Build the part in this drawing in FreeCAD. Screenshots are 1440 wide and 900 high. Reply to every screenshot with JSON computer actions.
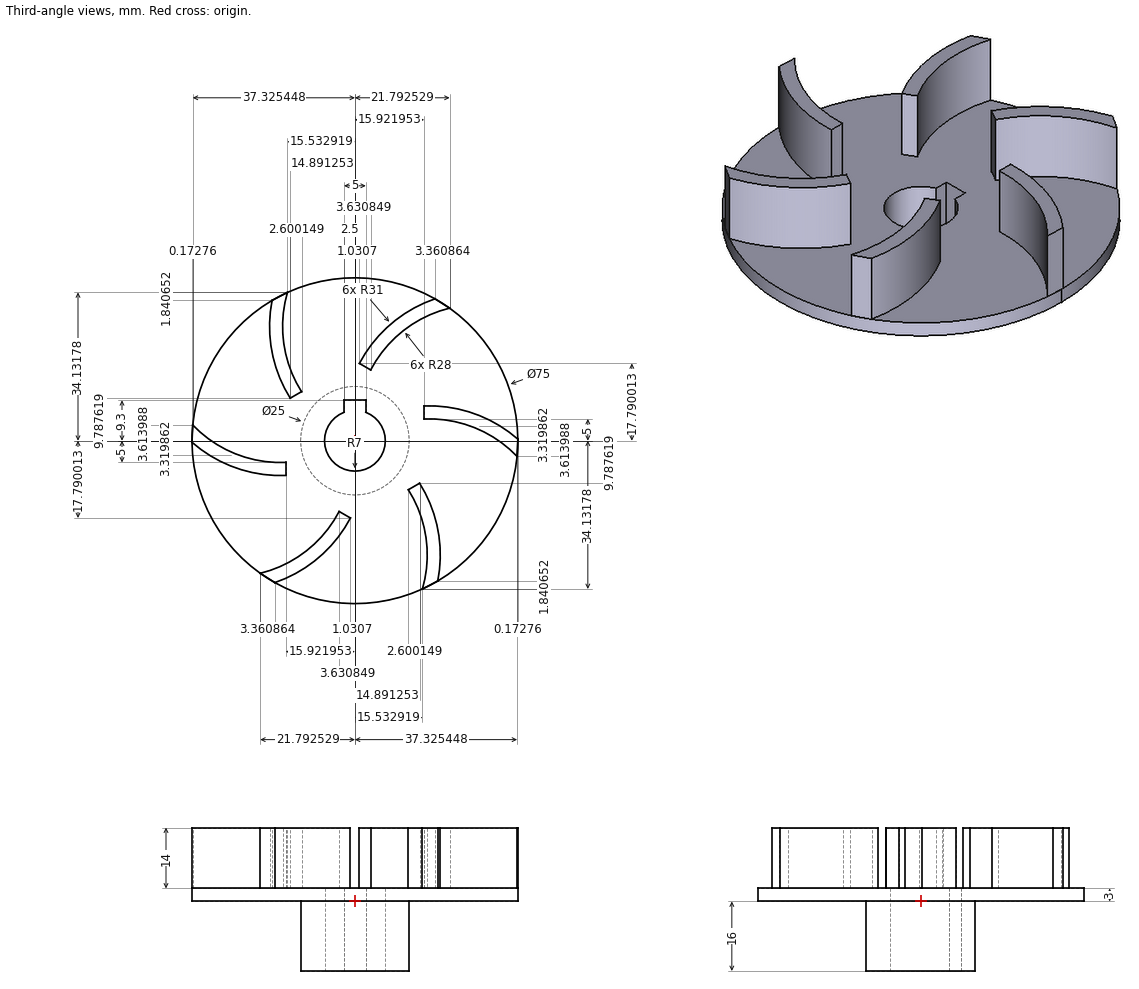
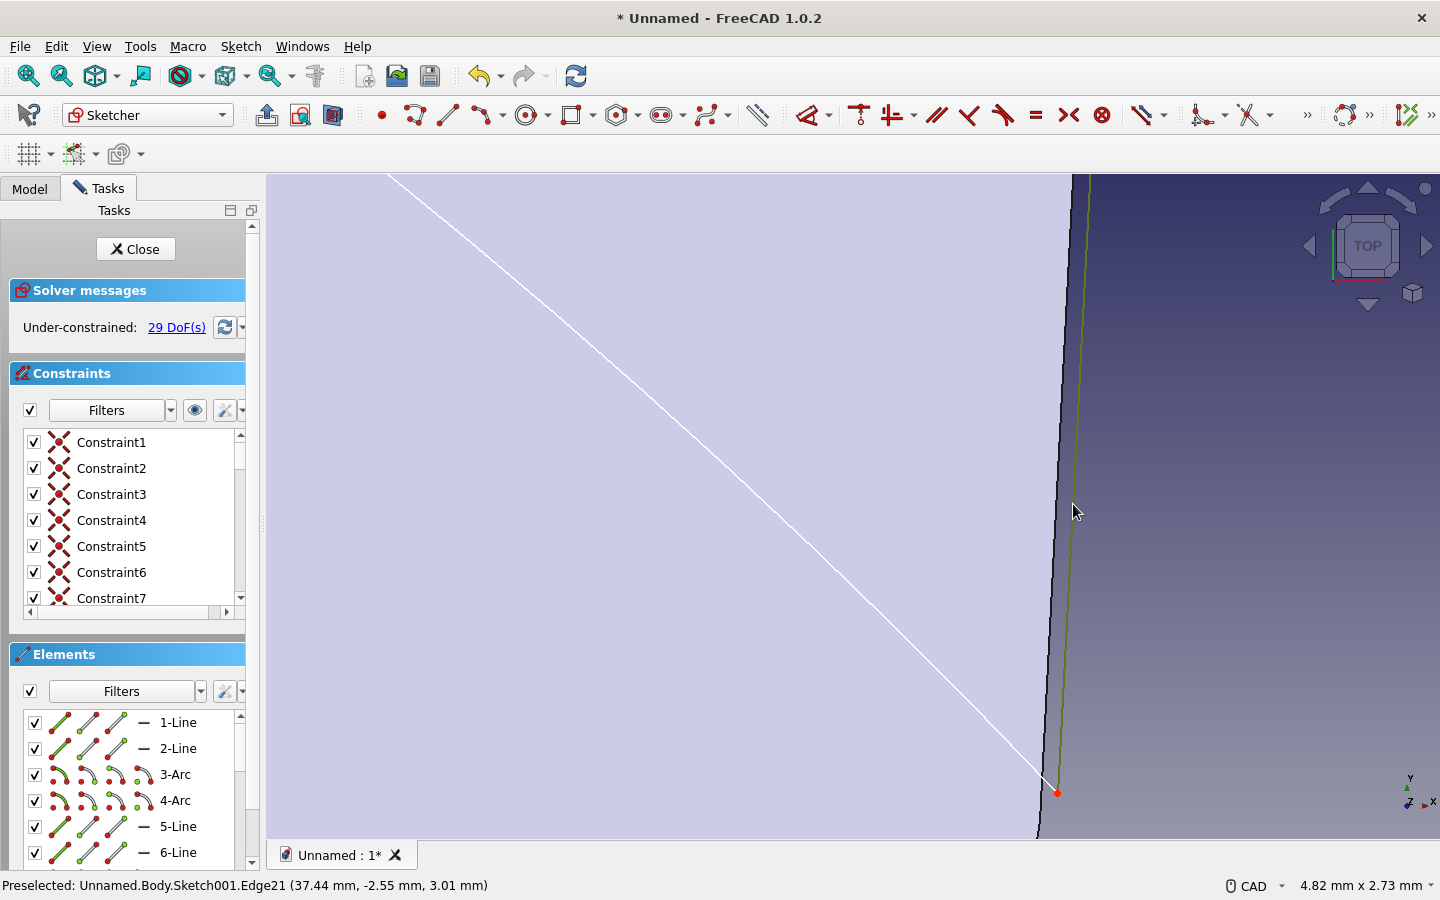
{"action": "key", "text": "l"}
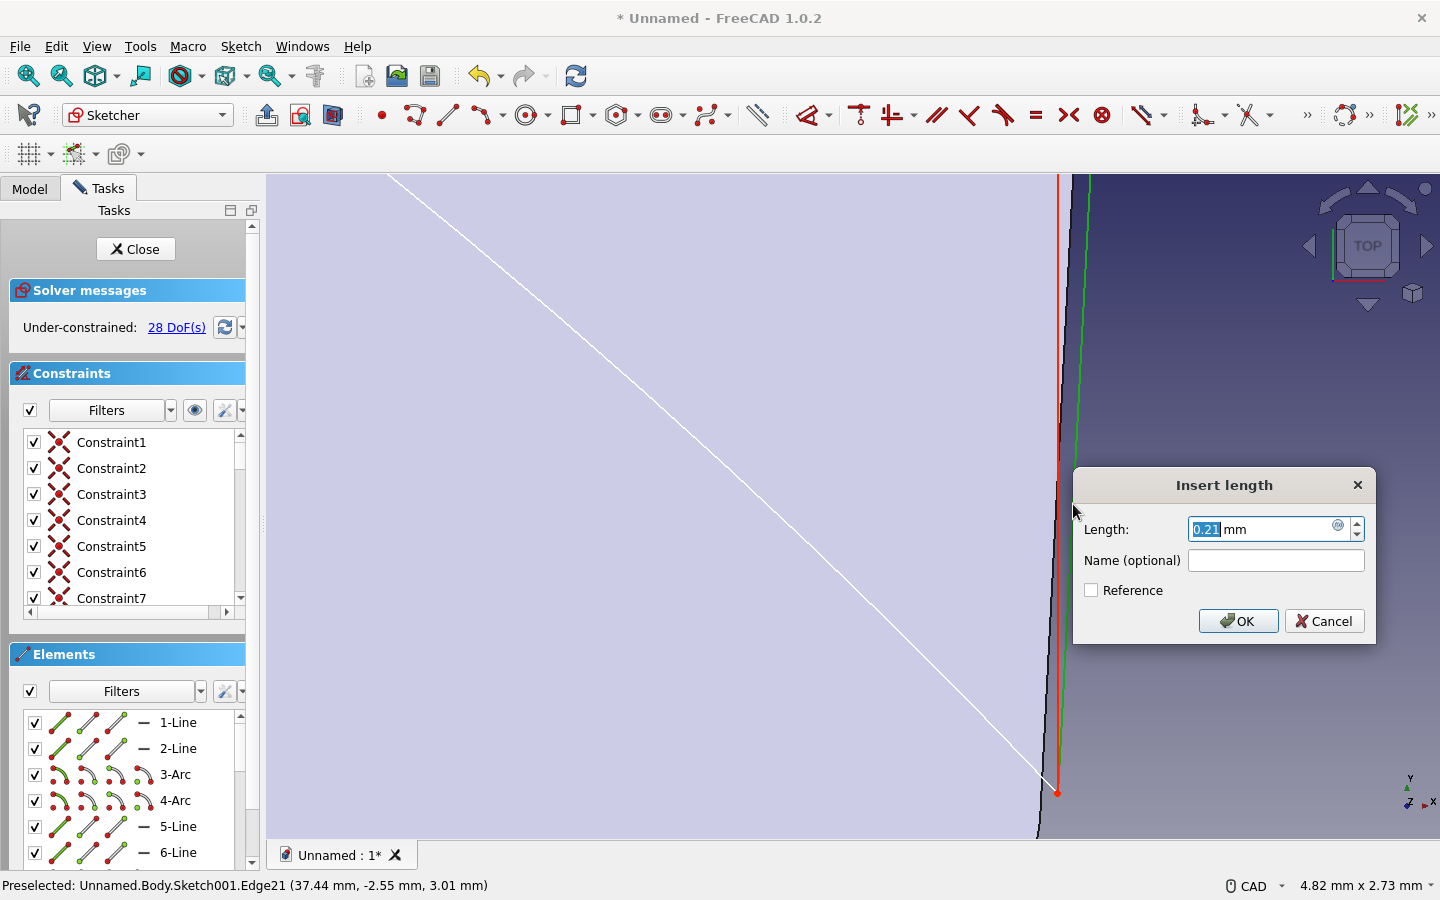
{"action": "type", "text": "0.17276"}
{"action": "key", "text": "Return"}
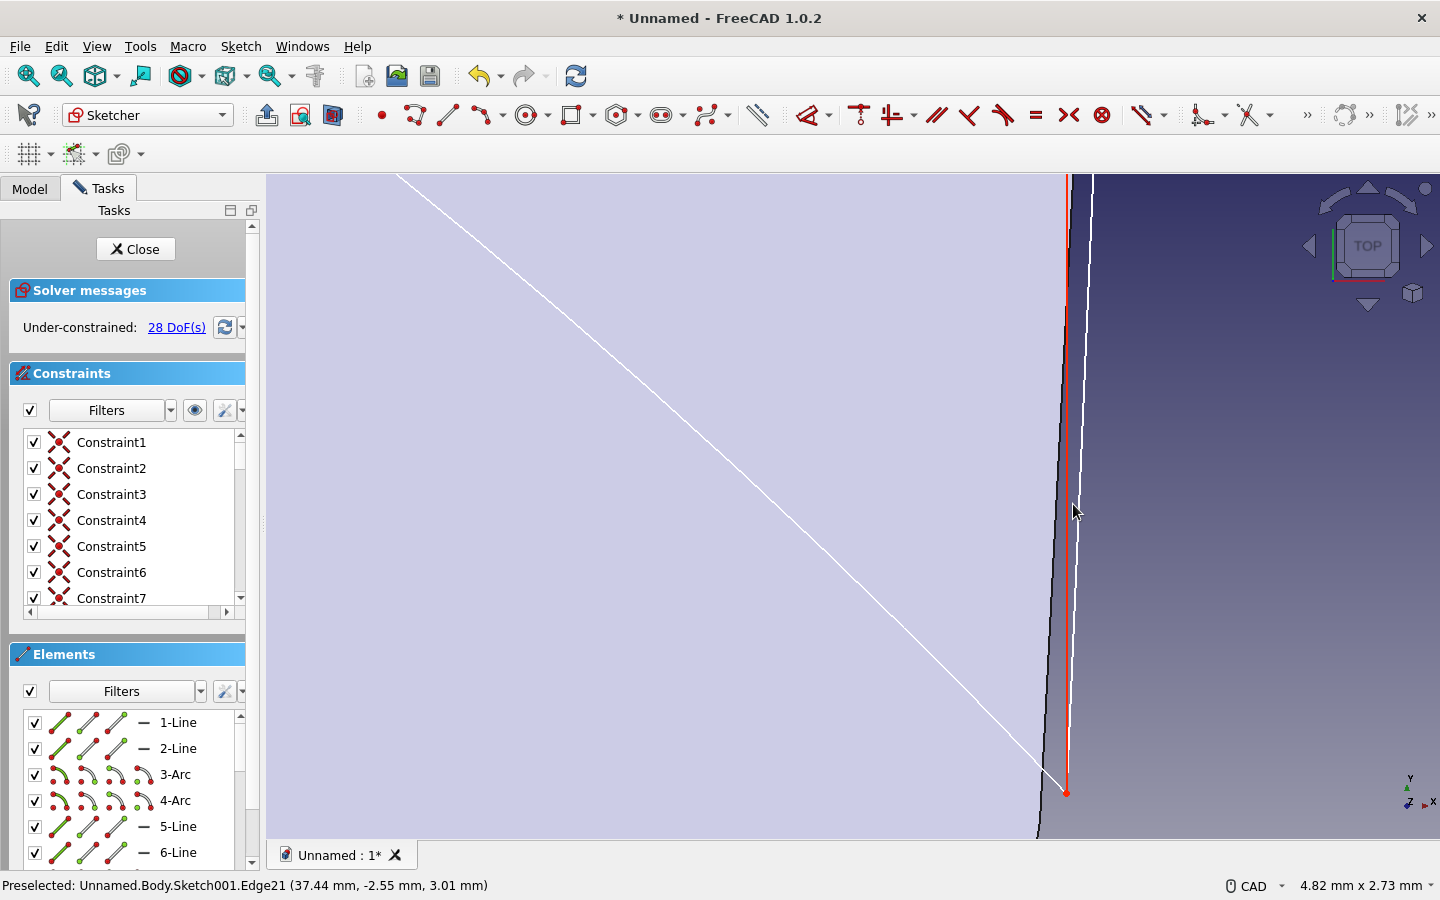
{"action": "scroll", "coordinate": [1089, 528], "scroll_direction": "down", "scroll_amount": 17}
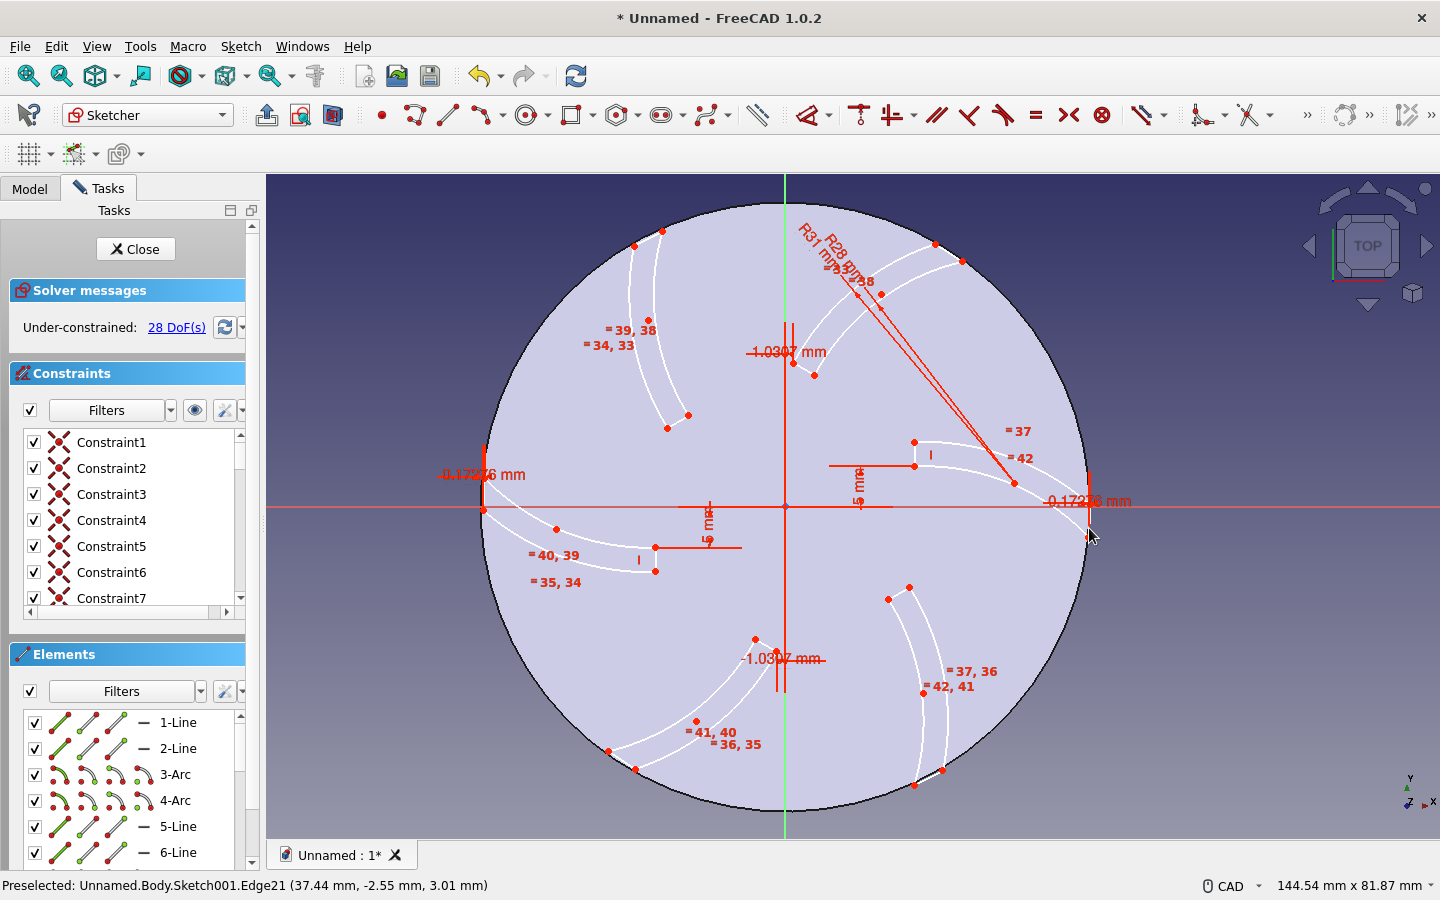
{"action": "scroll", "coordinate": [815, 375], "scroll_direction": "up", "scroll_amount": 2}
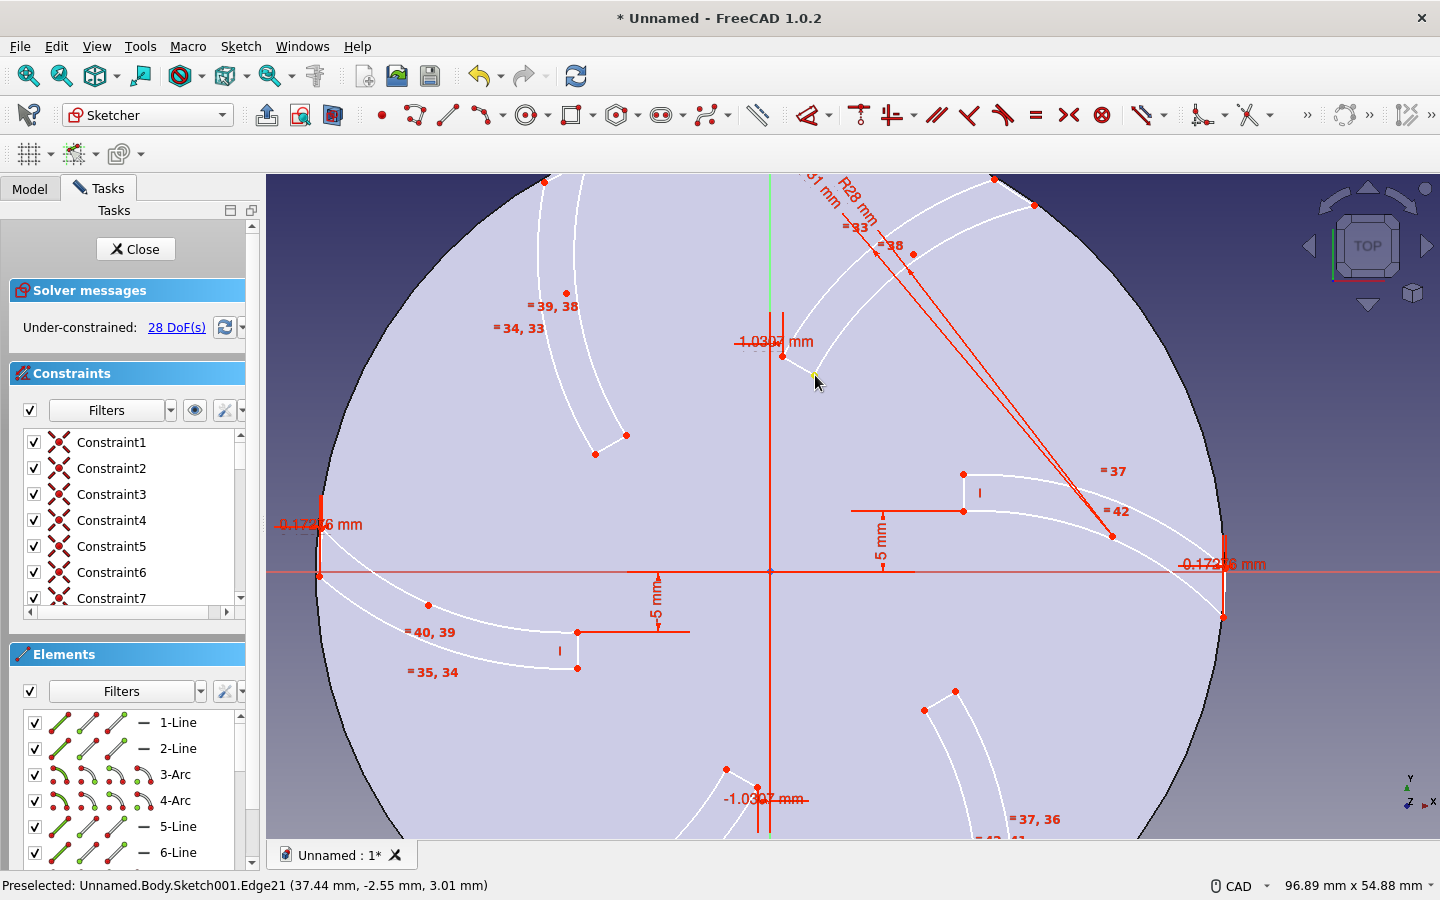
{"action": "left_click", "coordinate": [814, 375]}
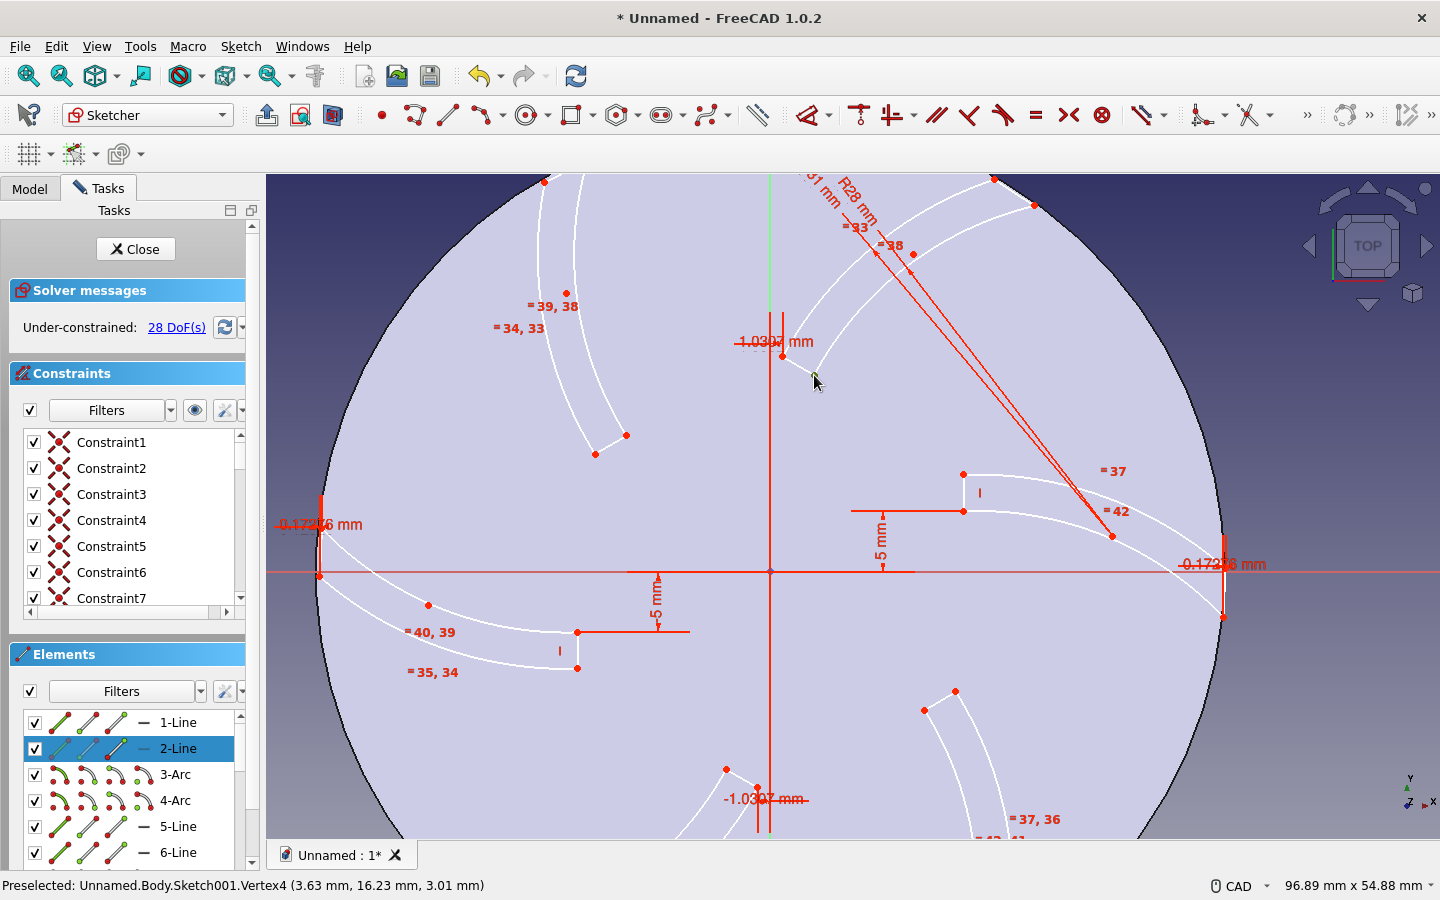
{"action": "key", "text": "l"}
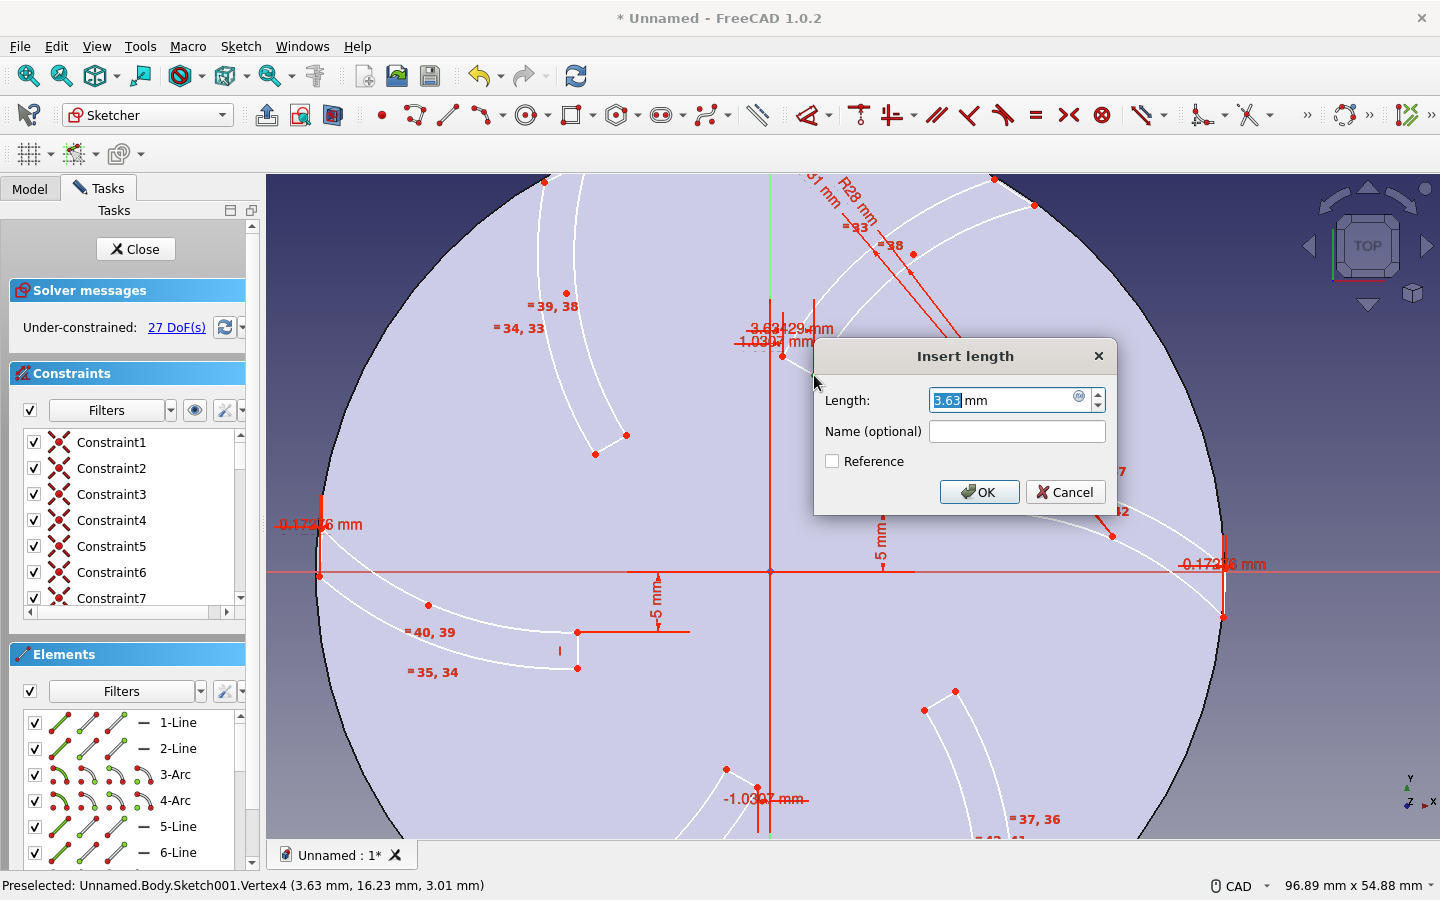
{"action": "type", "text": "3.630849"}
{"action": "key", "text": "Return"}